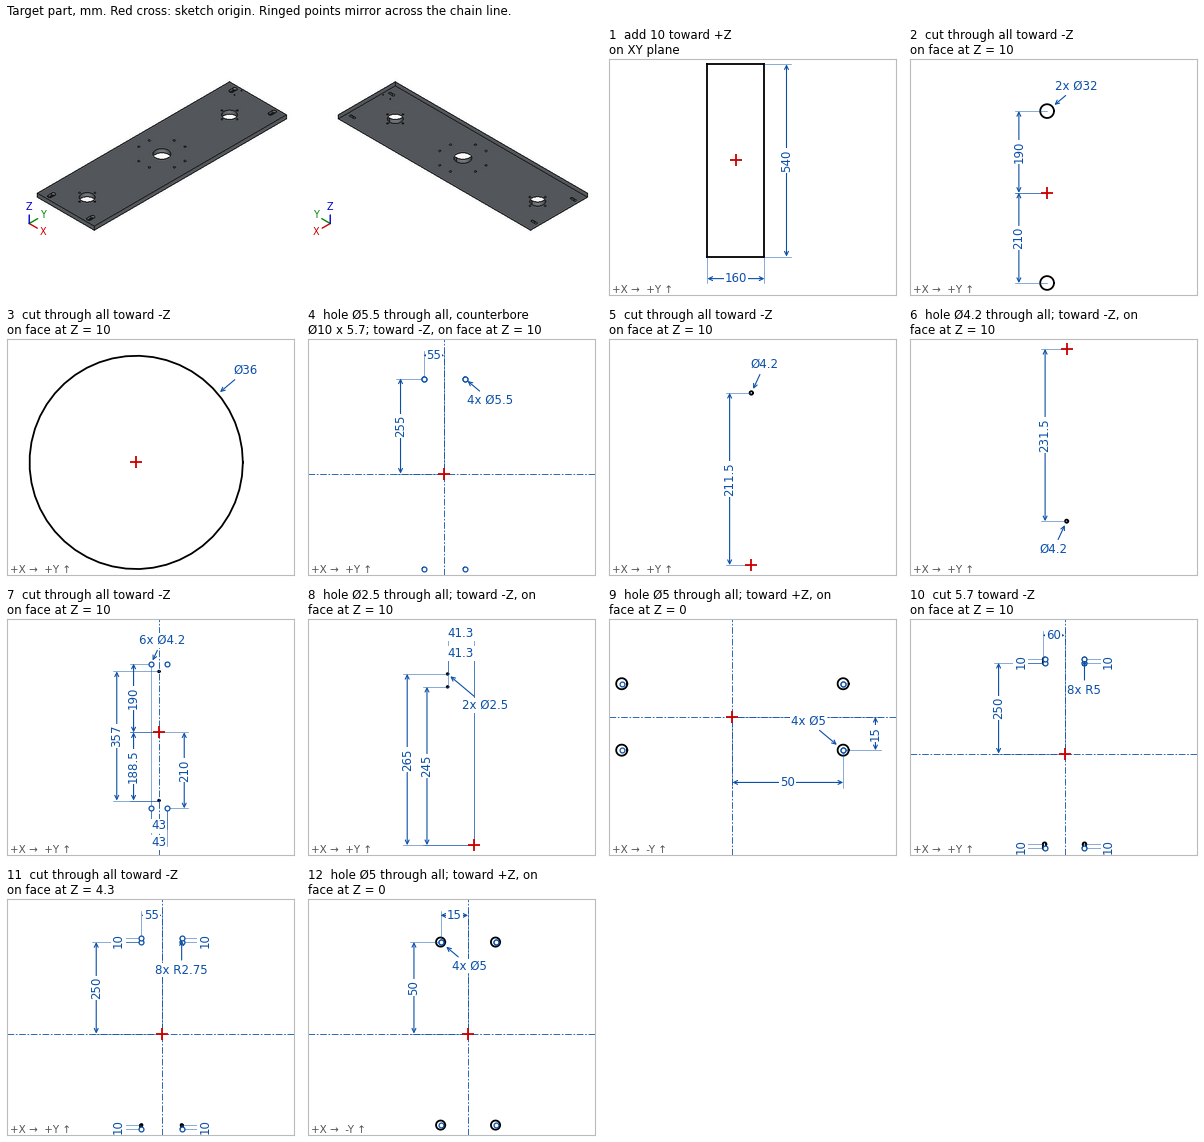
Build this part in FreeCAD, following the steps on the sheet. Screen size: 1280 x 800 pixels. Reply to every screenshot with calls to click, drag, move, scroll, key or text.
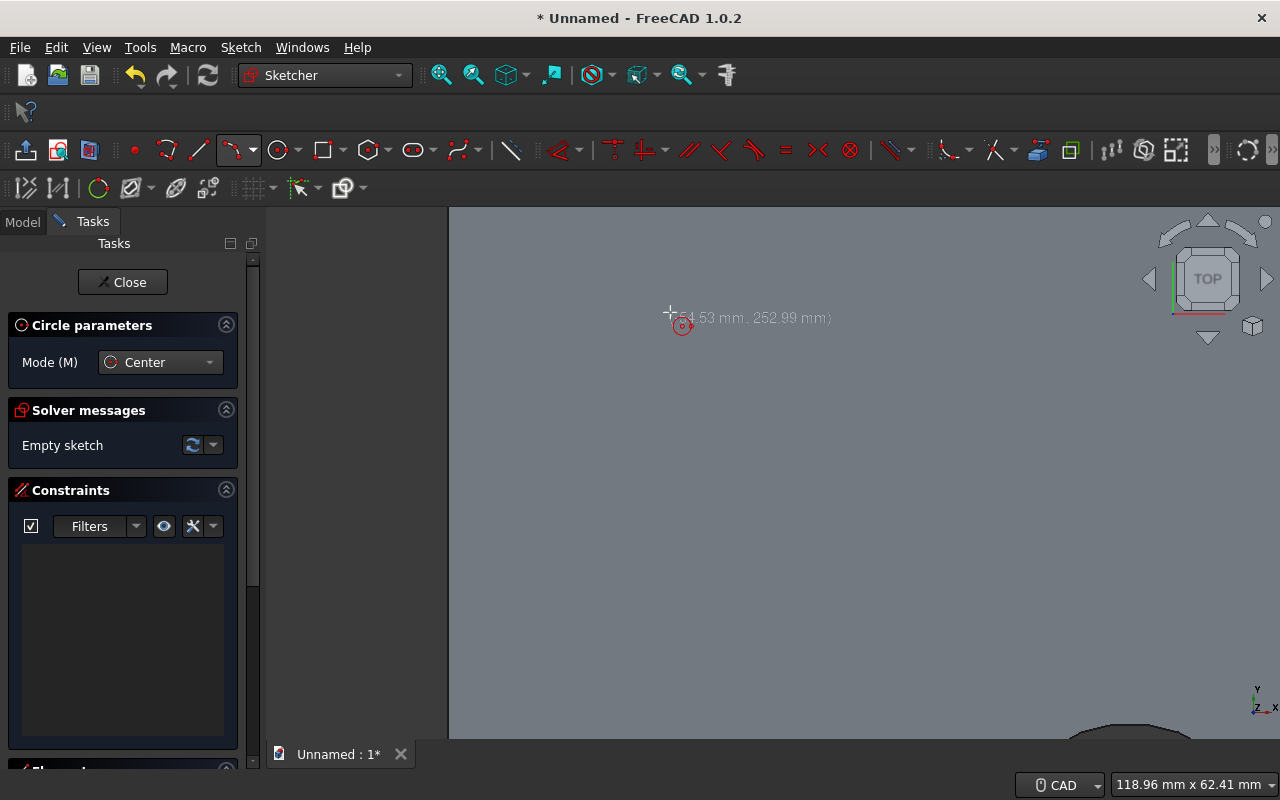
scroll(670, 312, down, 13)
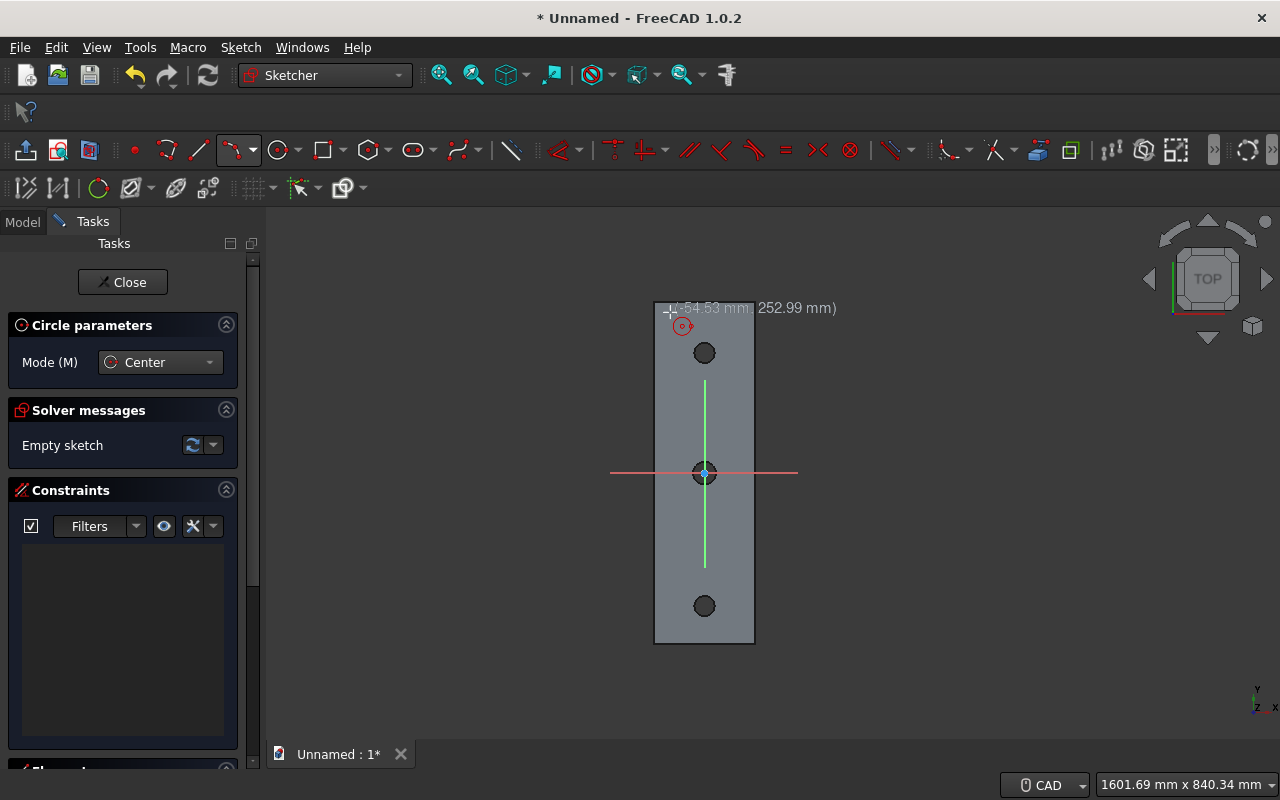
click(670, 312)
move(671, 310)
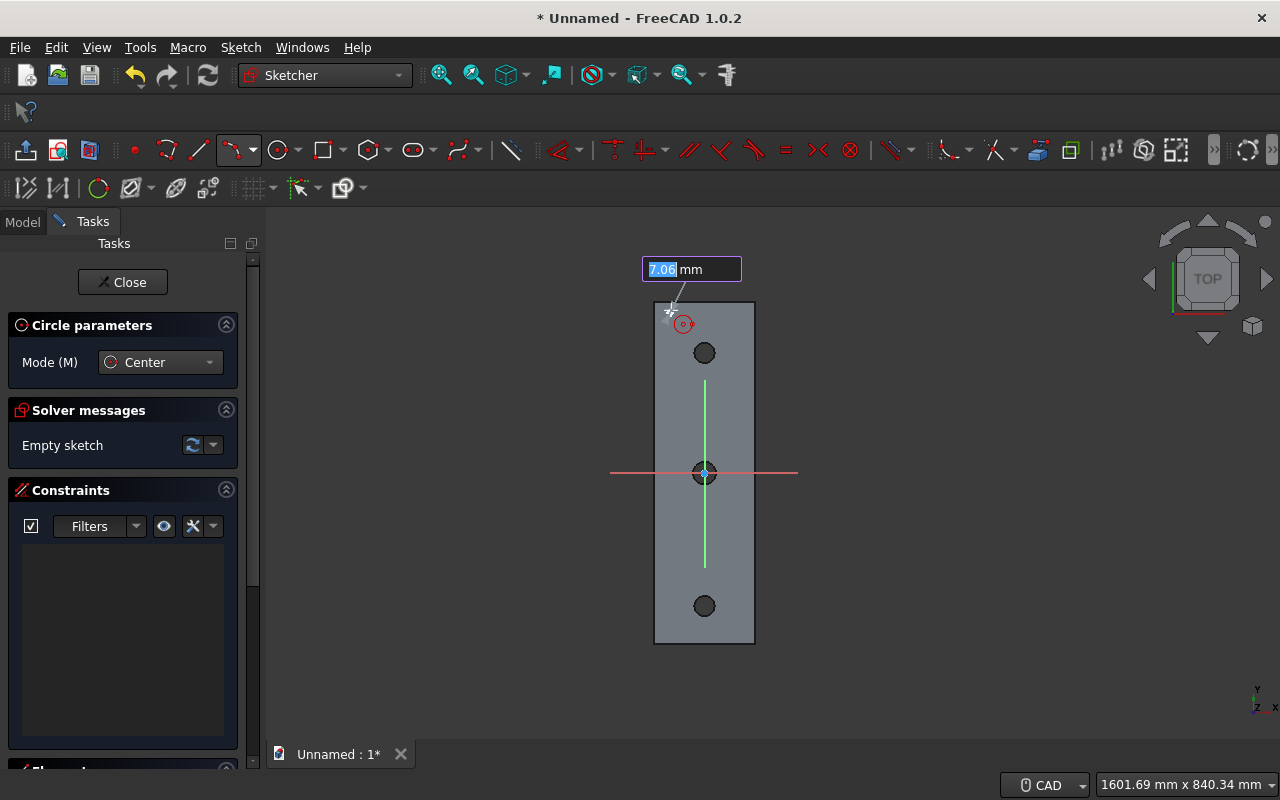
text(5.5)
key(Return)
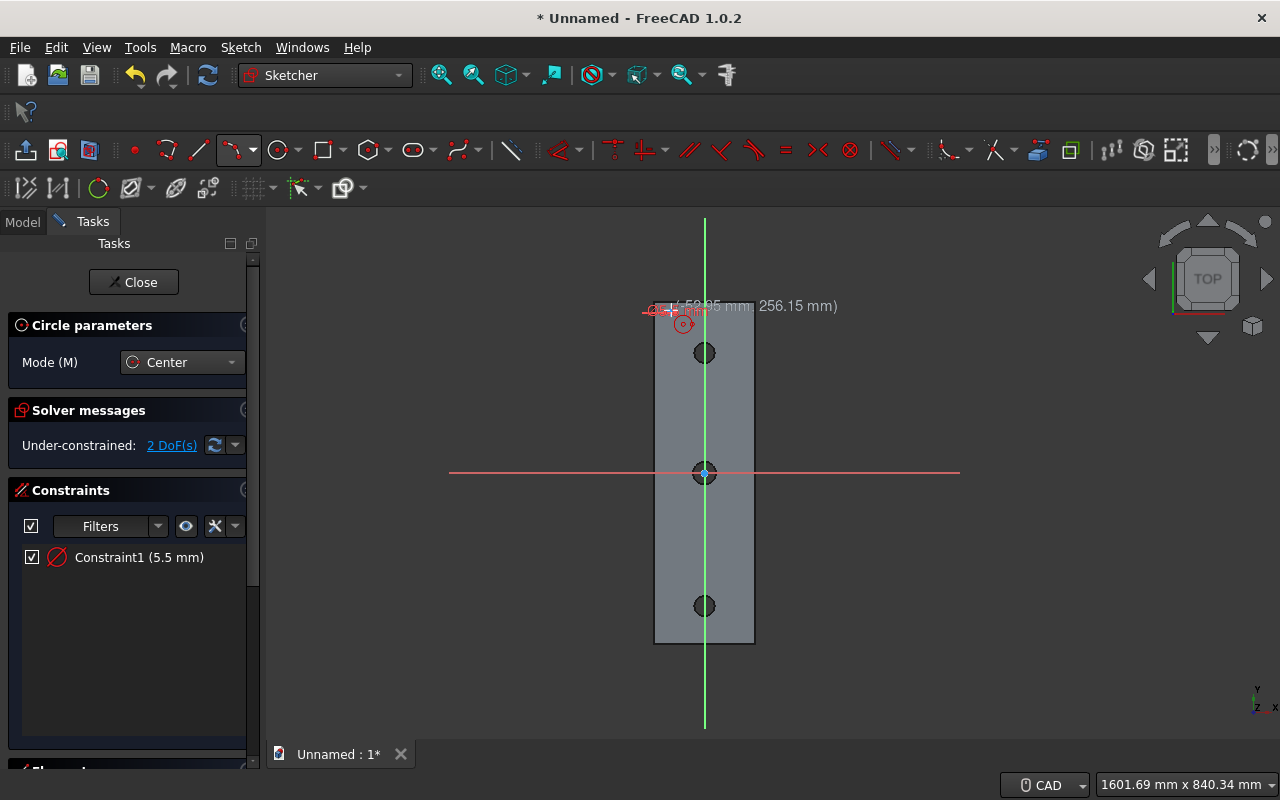
scroll(739, 312, up, 13)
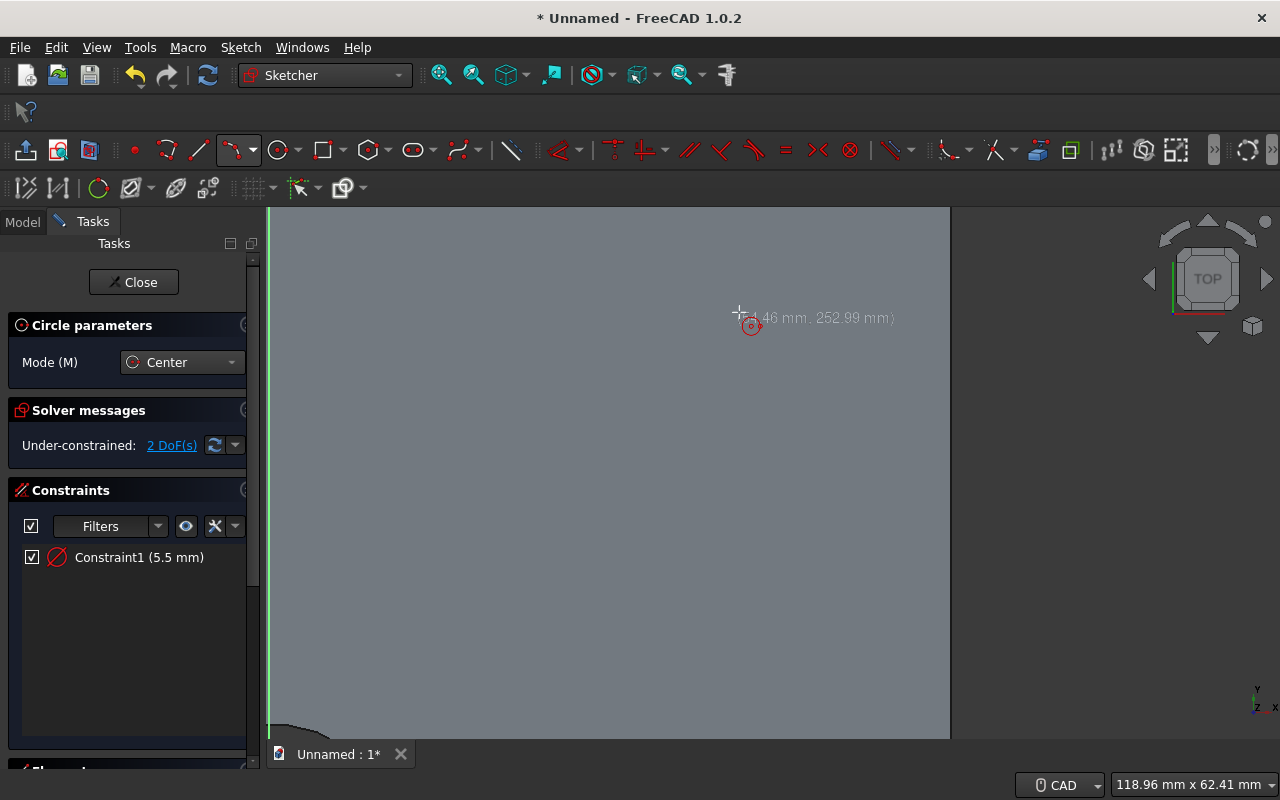
scroll(739, 312, down, 13)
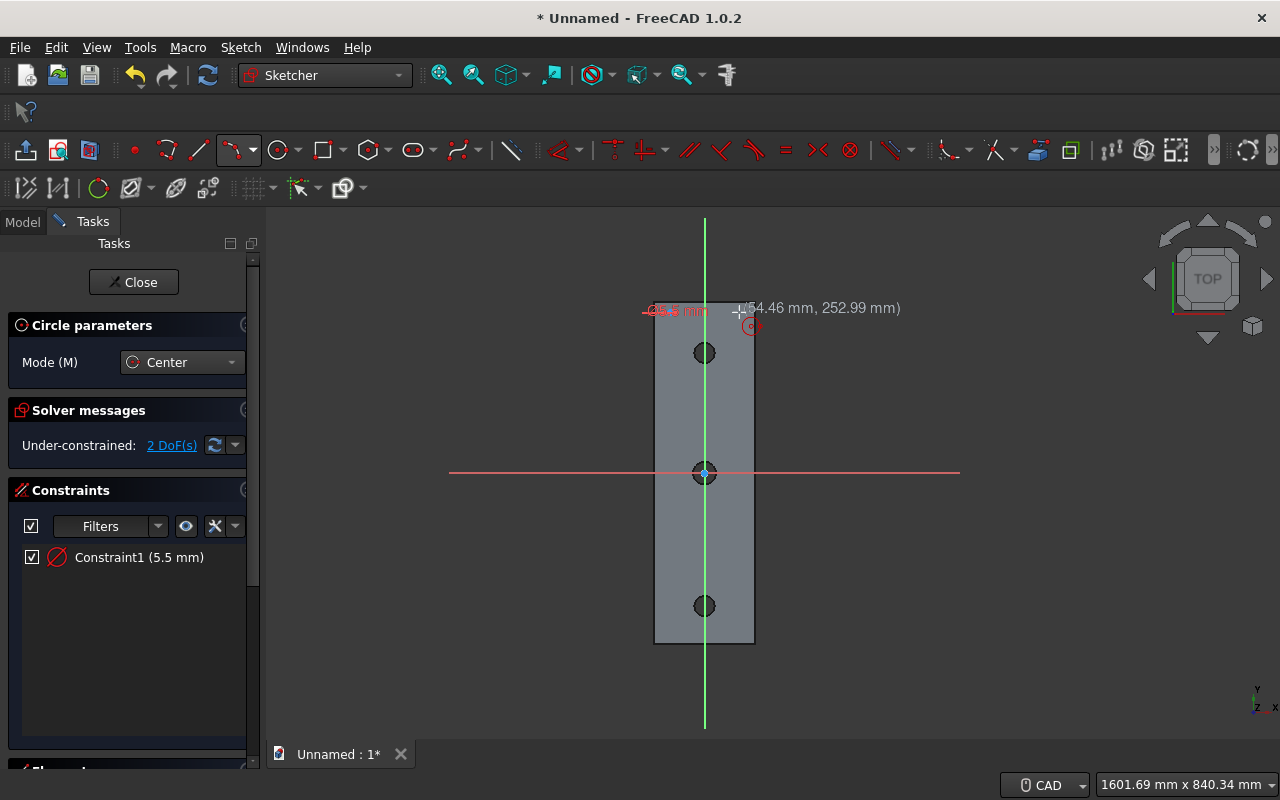
click(739, 312)
move(741, 310)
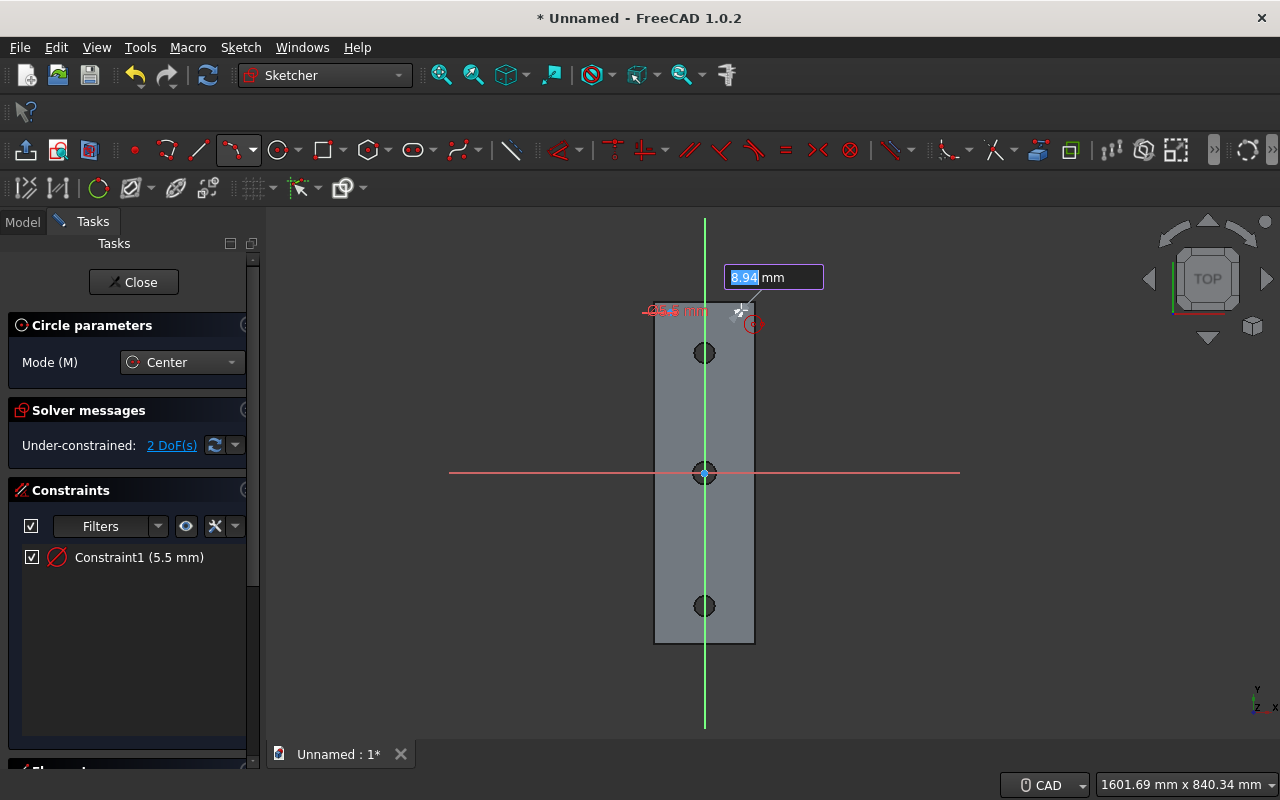
text(5.5)
key(Return)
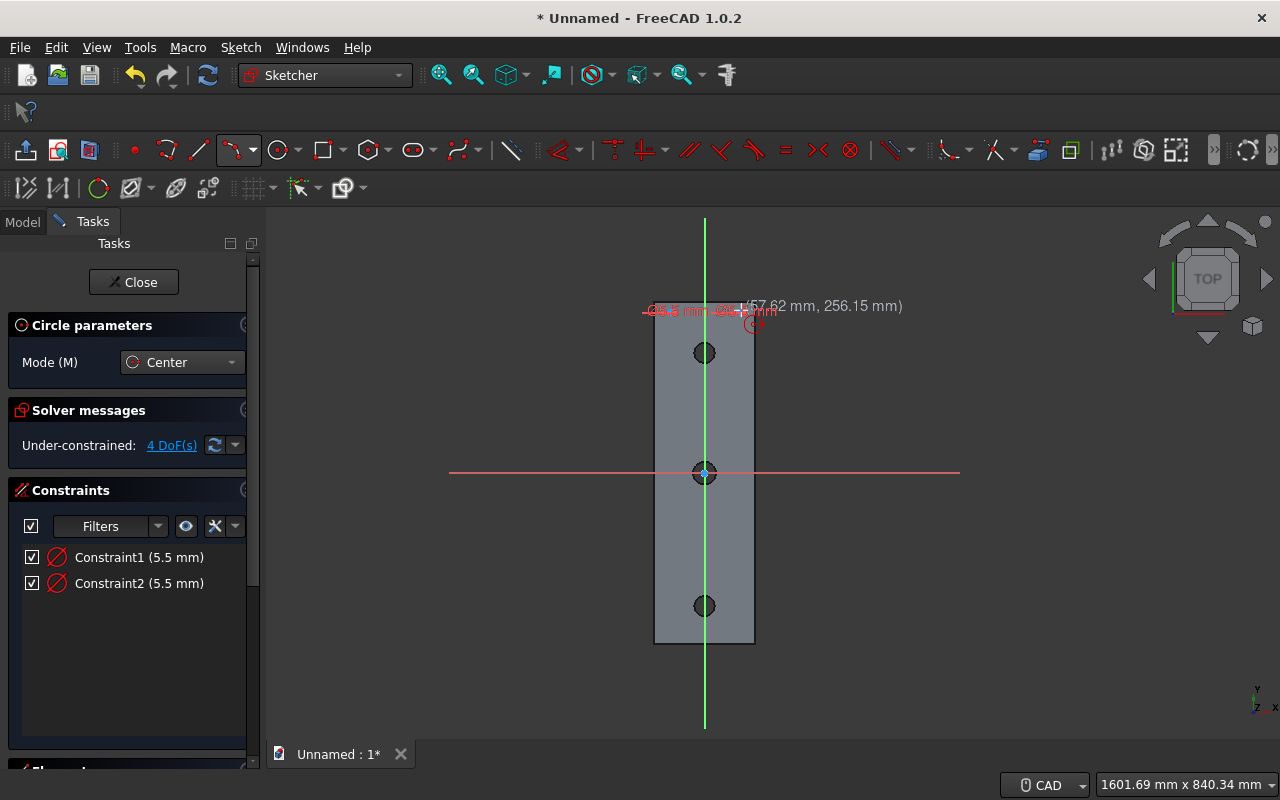
scroll(739, 635, up, 13)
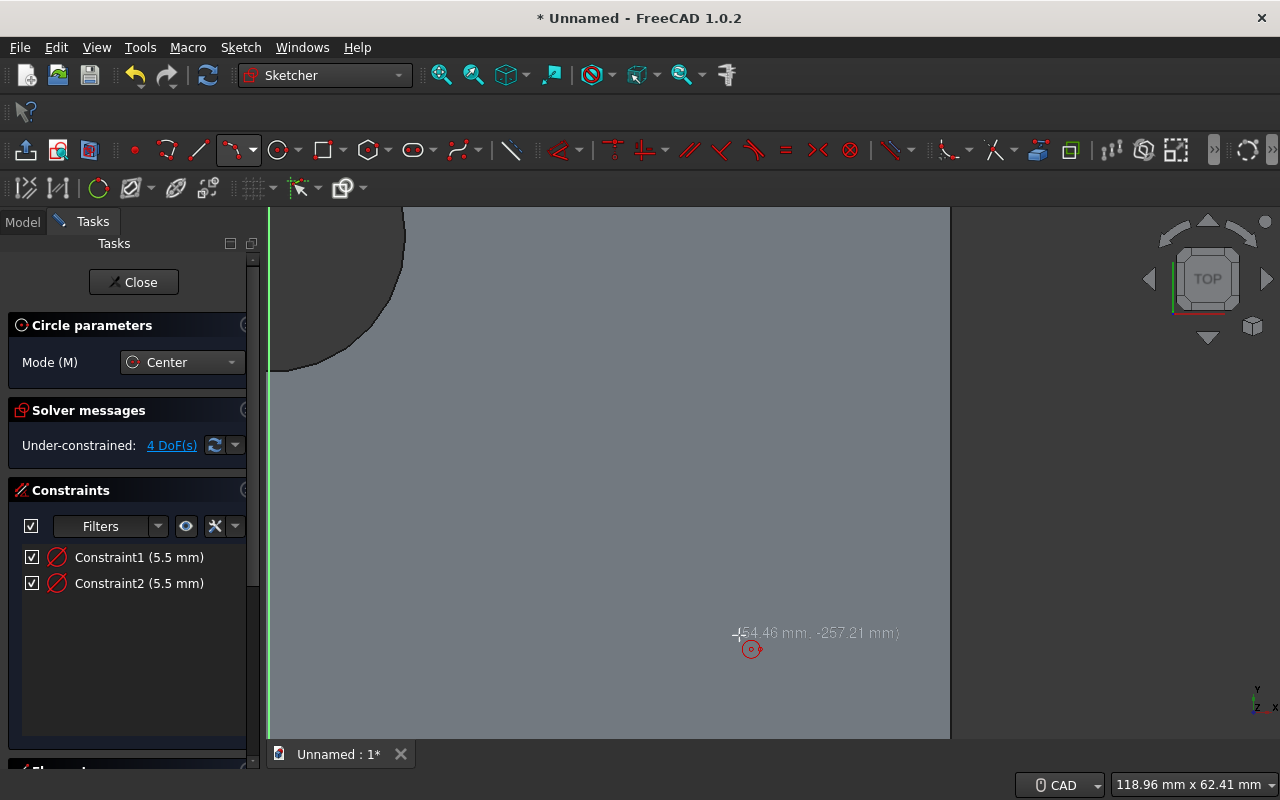
scroll(739, 636, down, 13)